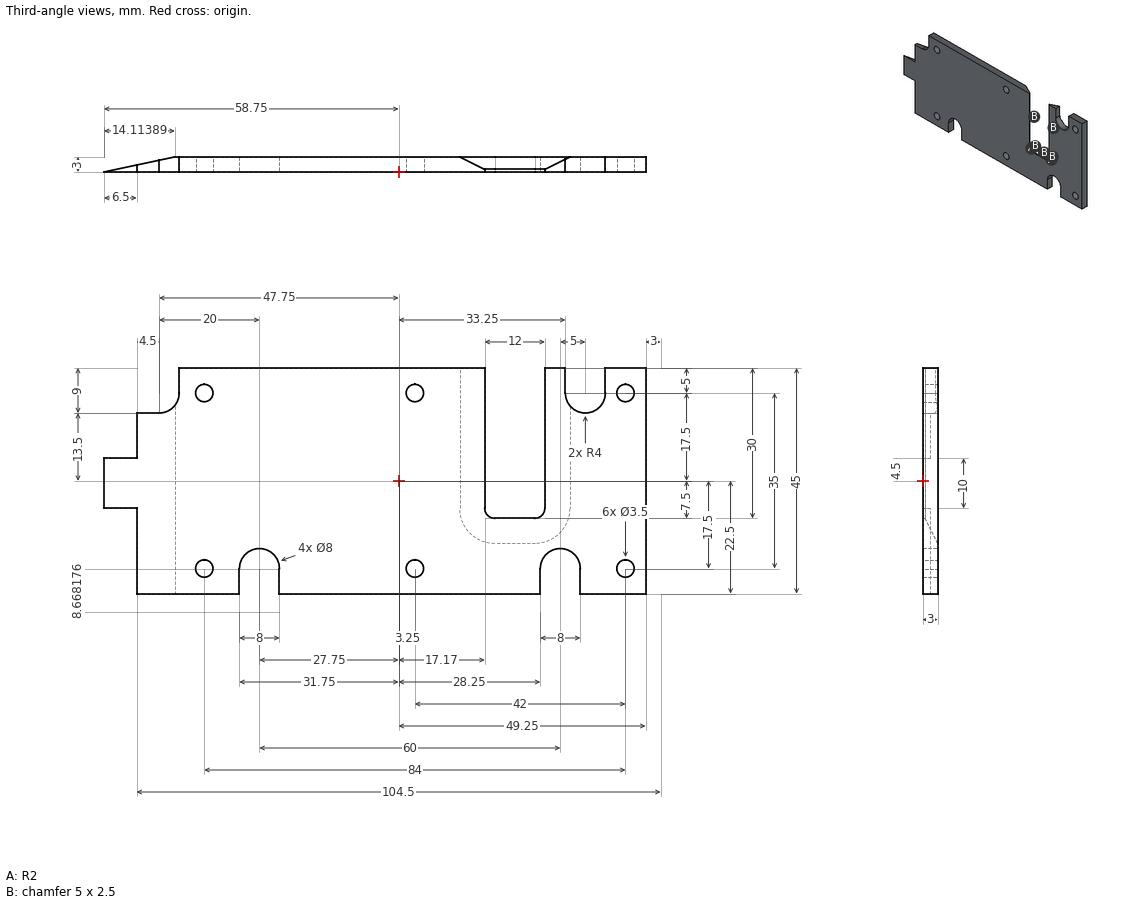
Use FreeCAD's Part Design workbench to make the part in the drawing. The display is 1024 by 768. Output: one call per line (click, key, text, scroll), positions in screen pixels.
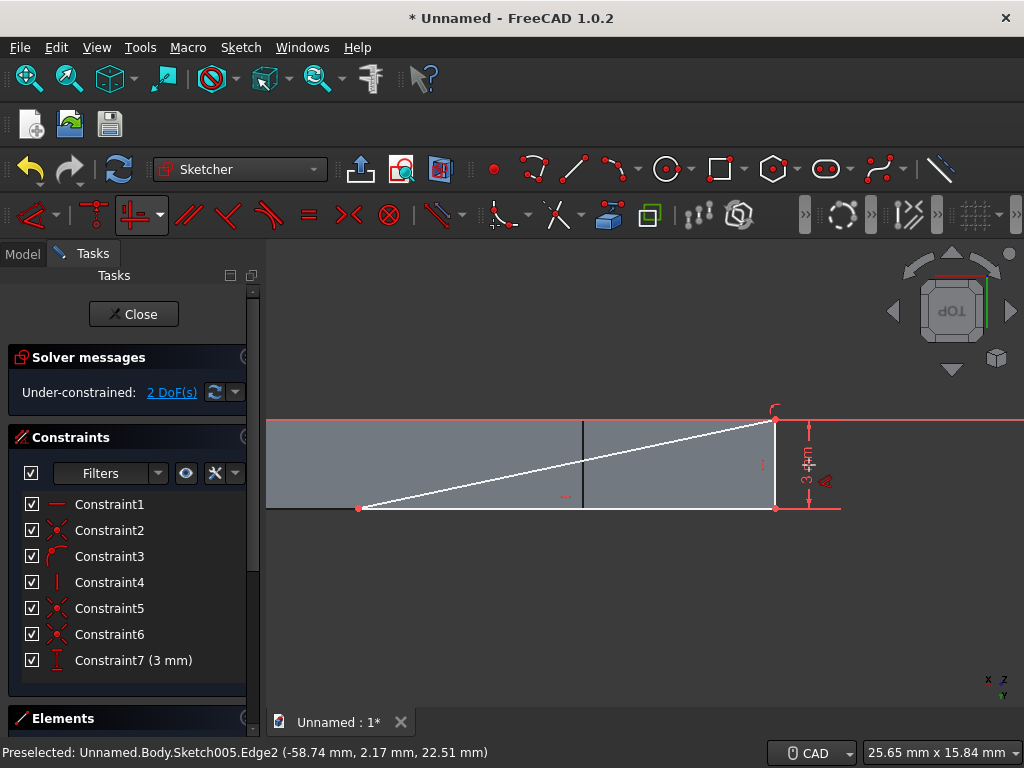
click(775, 509)
click(535, 543)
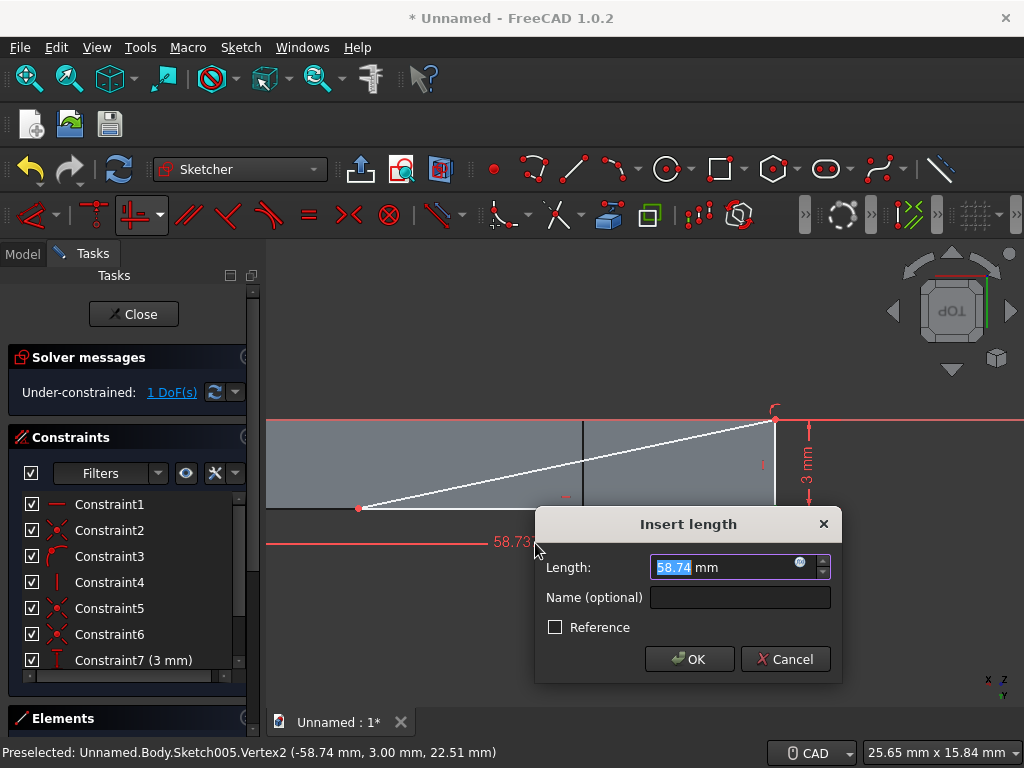
text(58.75)
key(Return)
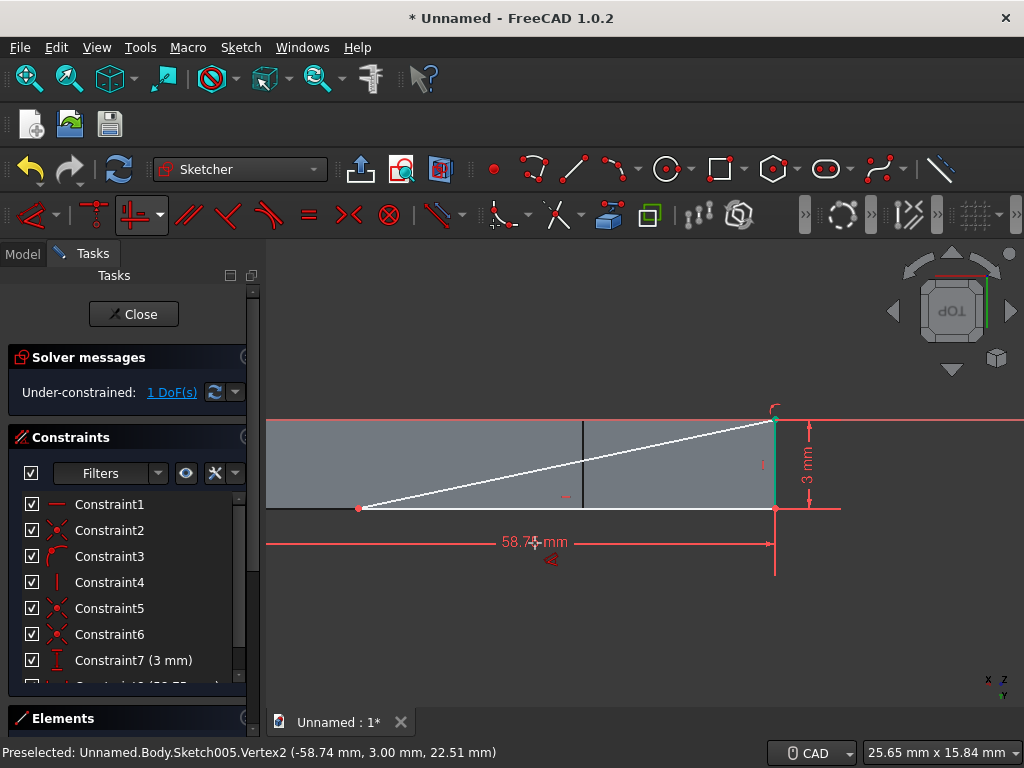
click(483, 509)
click(663, 543)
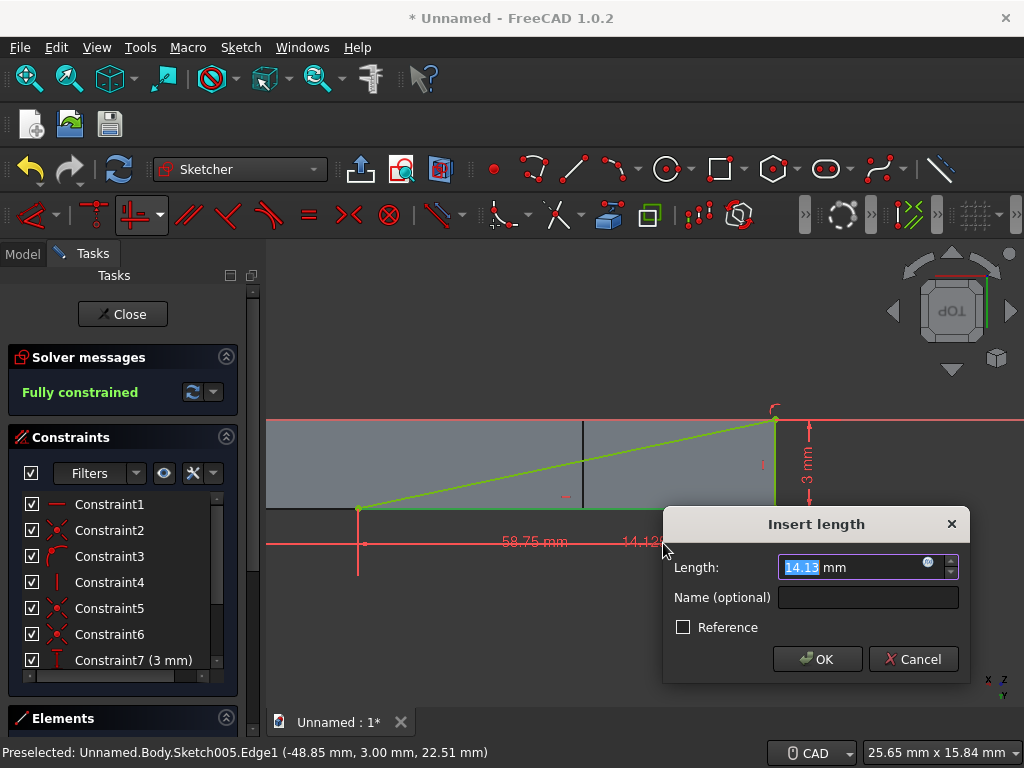
text(14.11389)
key(Return)
key(Escape)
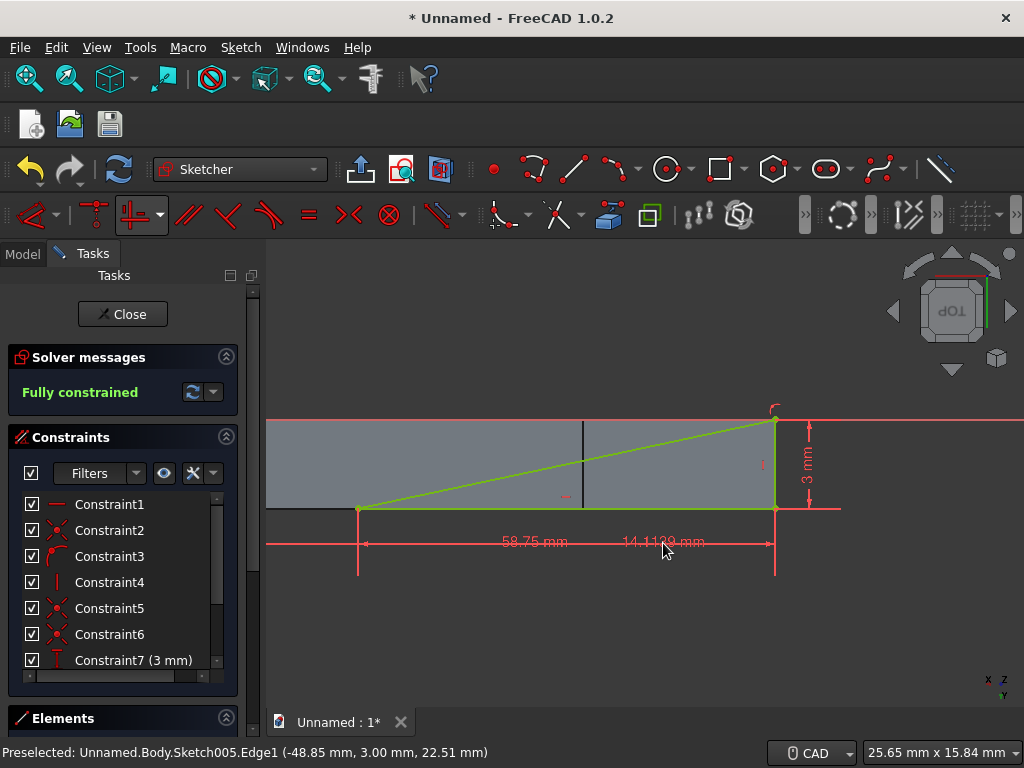
click(123, 314)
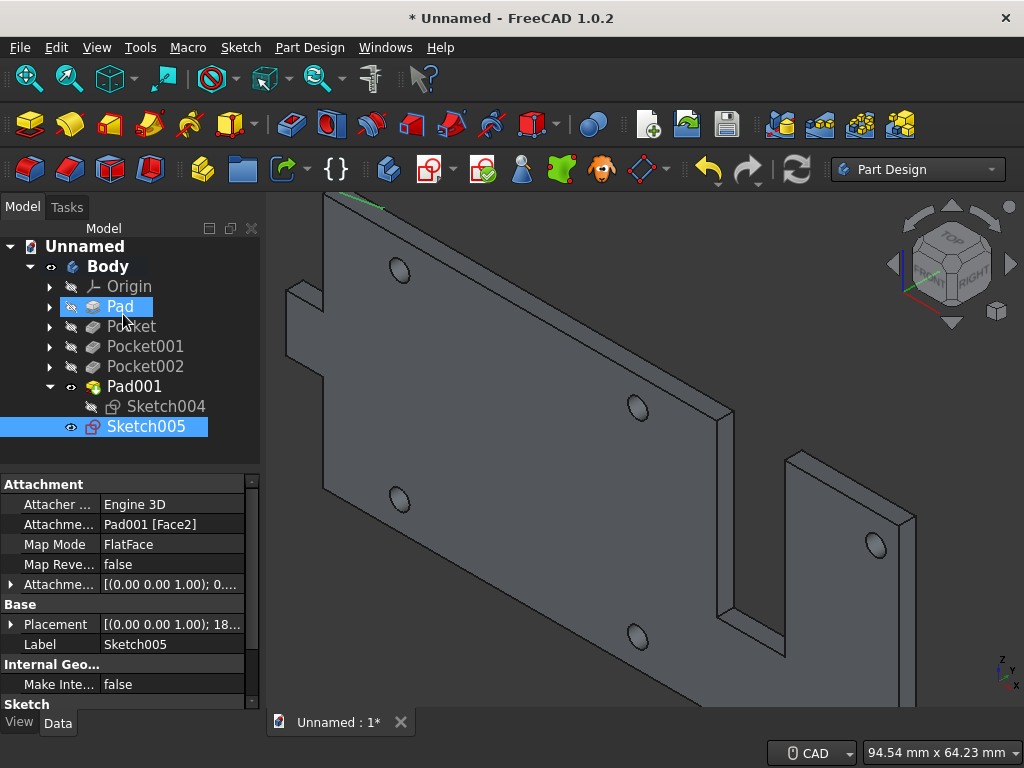
click(292, 124)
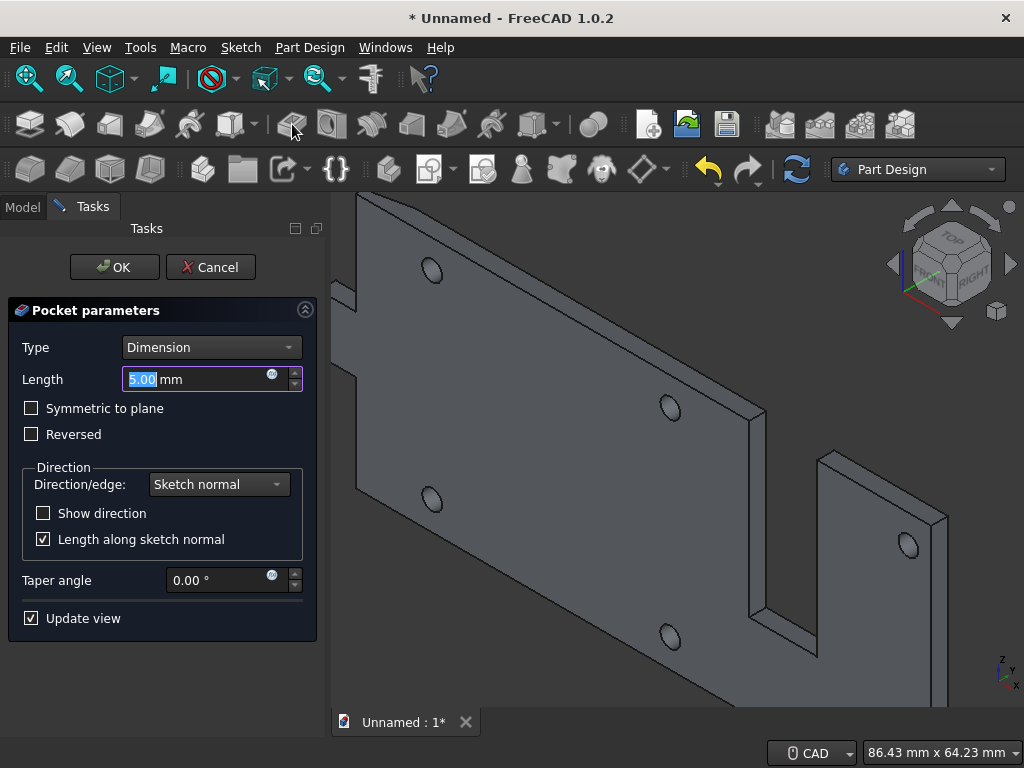
click(212, 348)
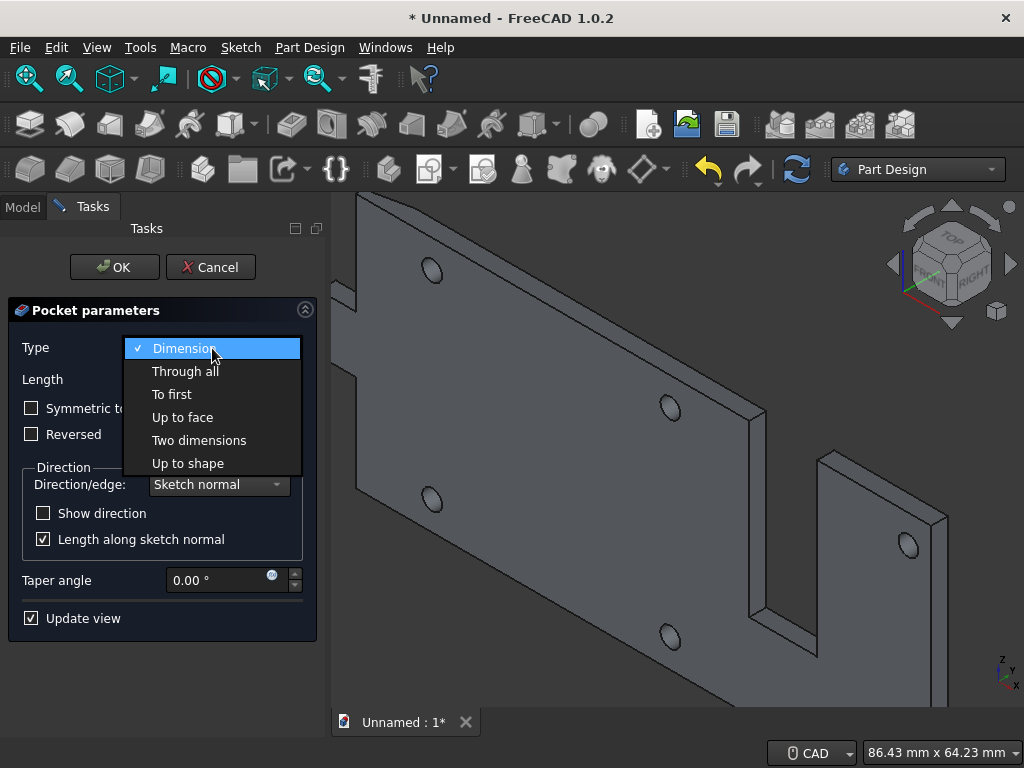
click(212, 372)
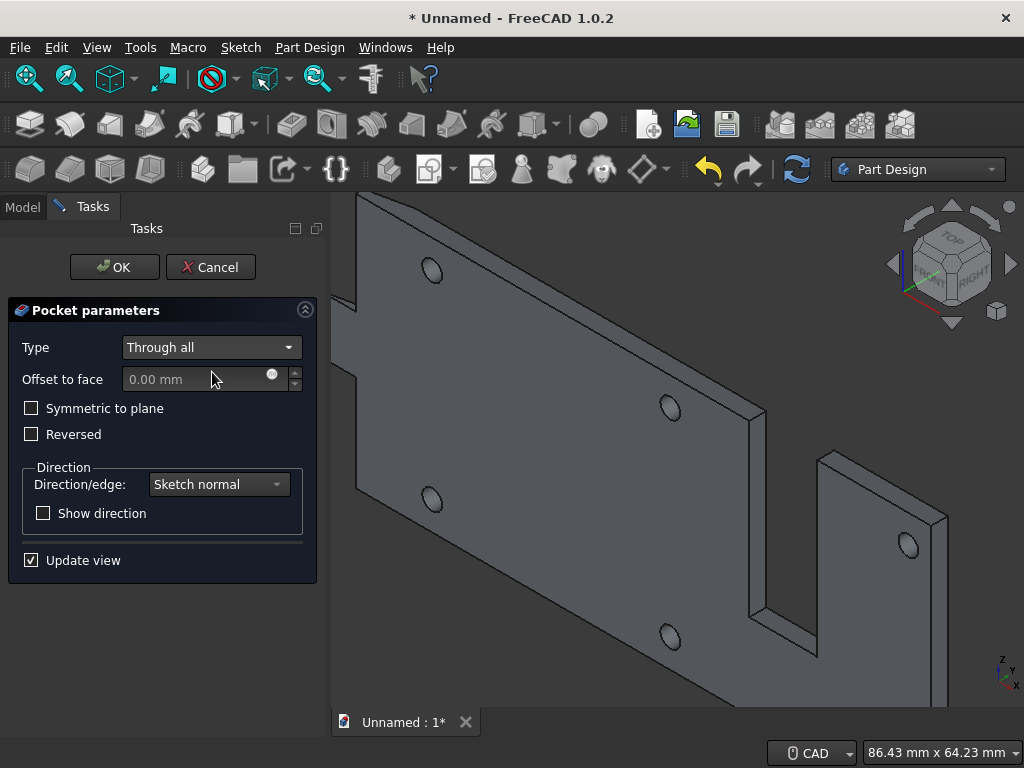
click(115, 267)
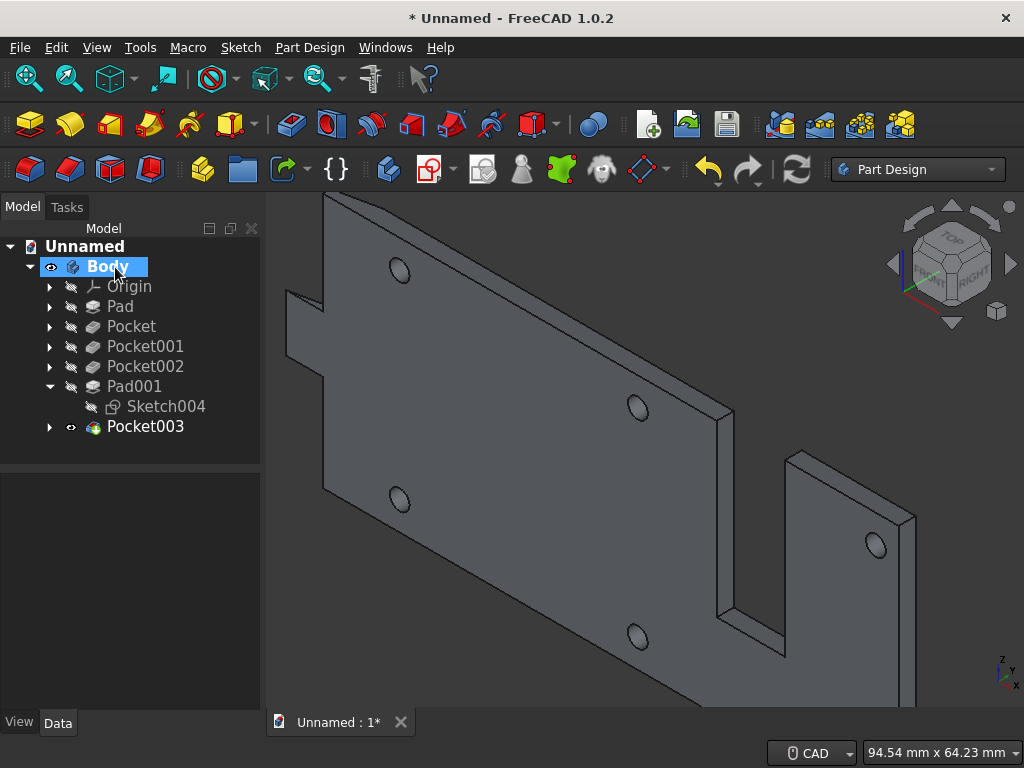
key(v)
key(f)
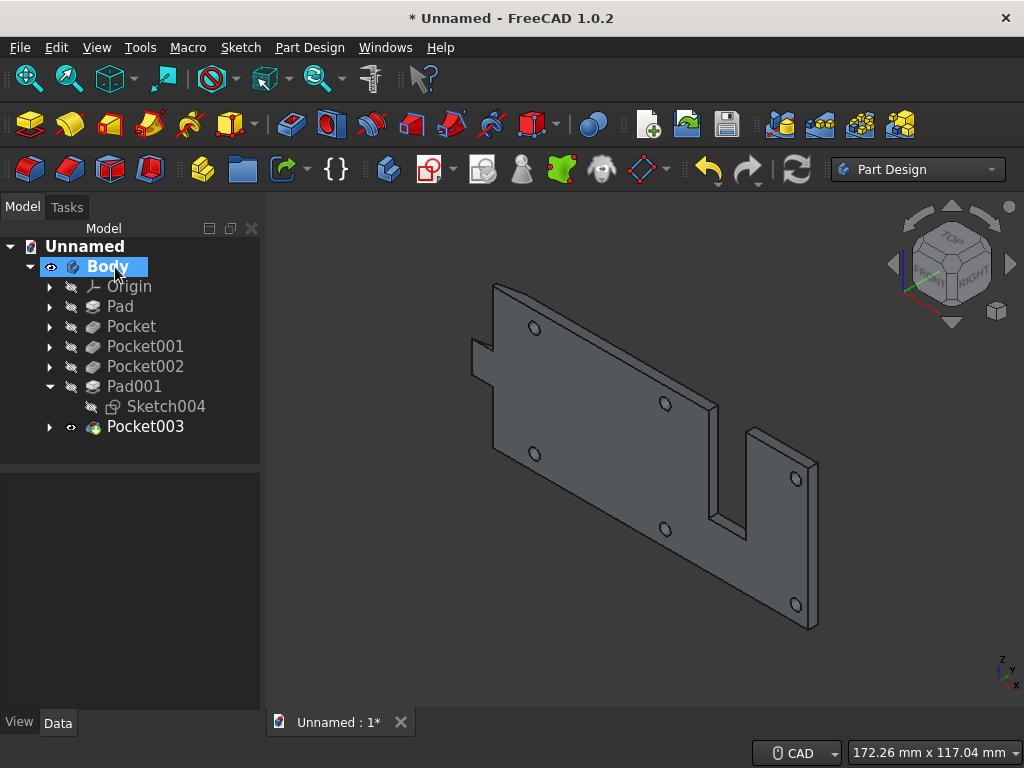
key(4)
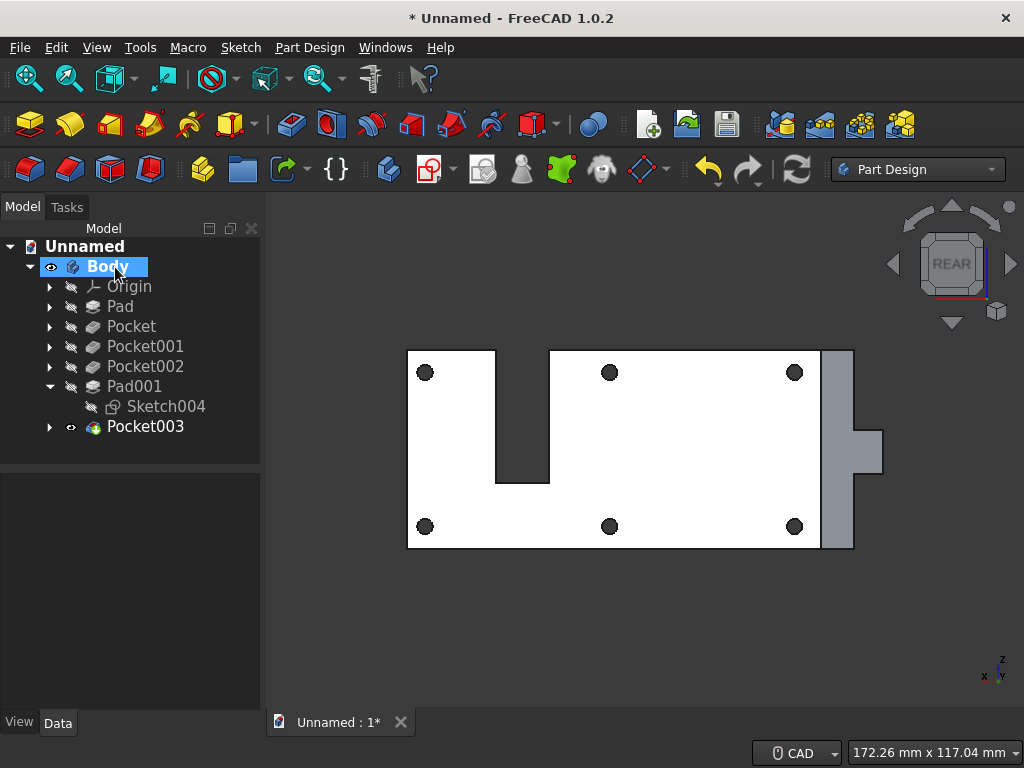
click(673, 448)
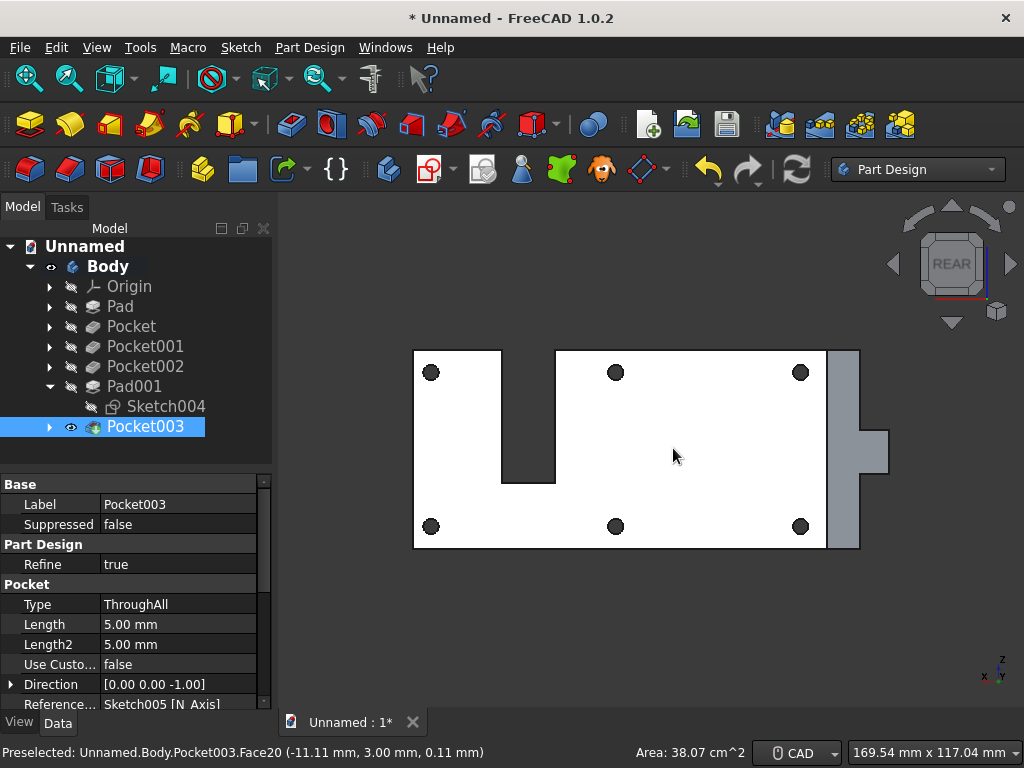
click(430, 170)